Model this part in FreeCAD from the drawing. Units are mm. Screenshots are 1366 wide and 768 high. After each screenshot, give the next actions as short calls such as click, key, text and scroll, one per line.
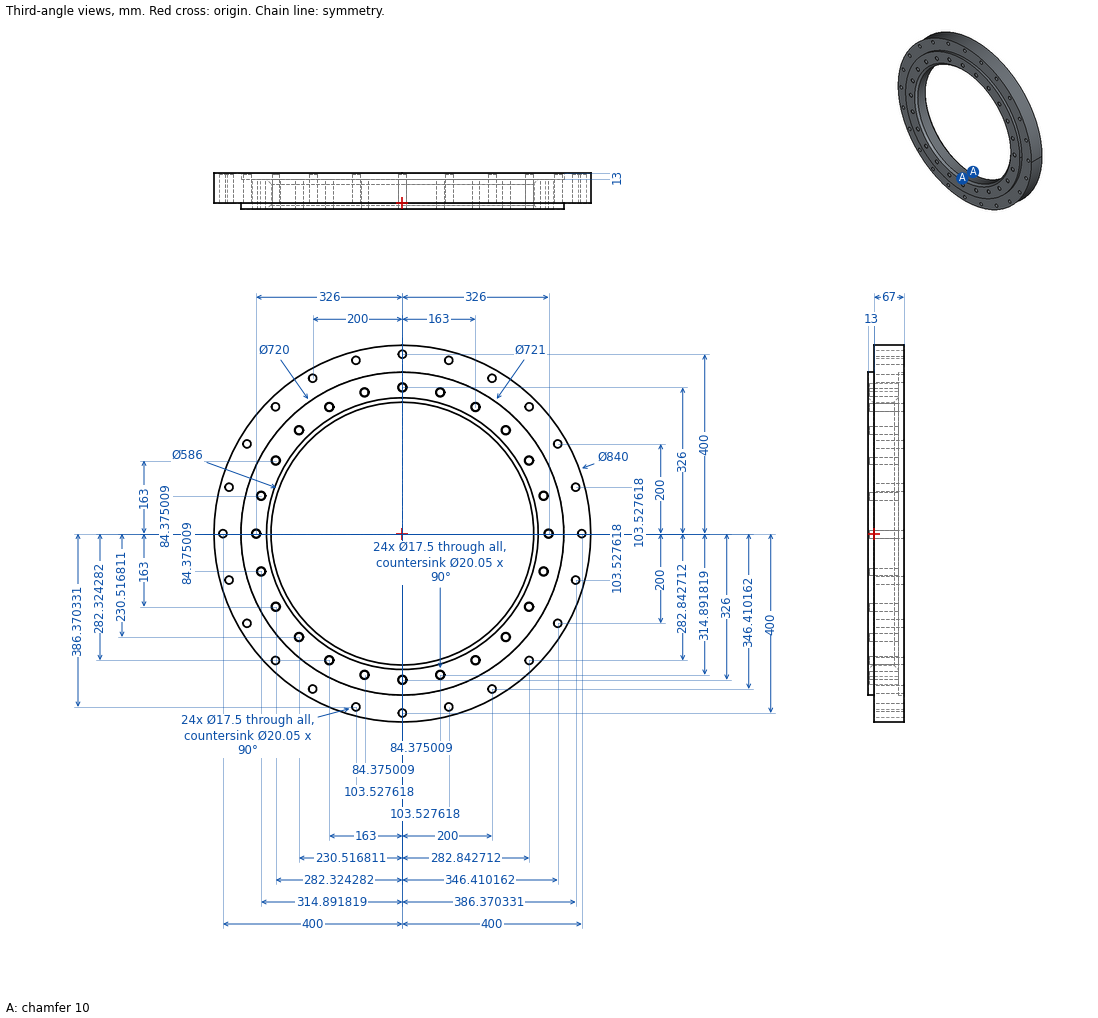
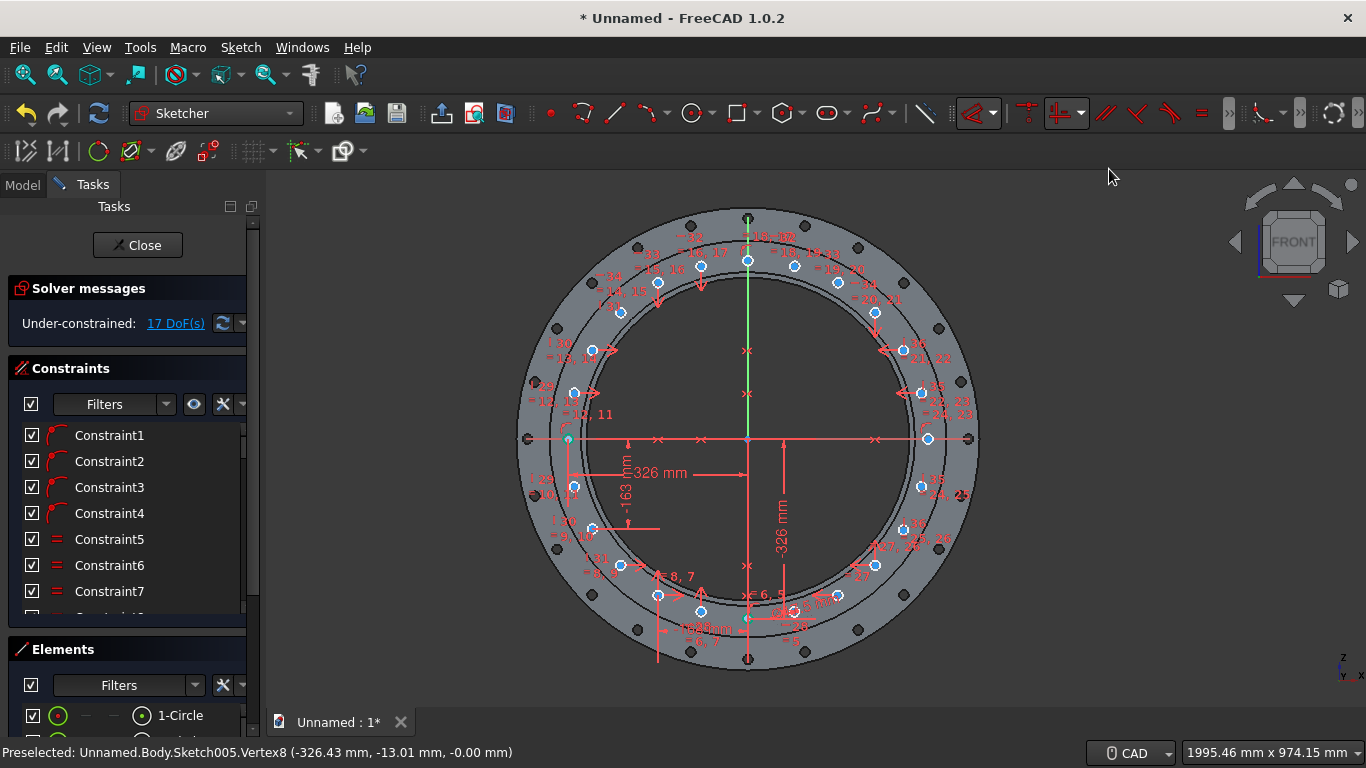
scroll(592, 350, up, 4)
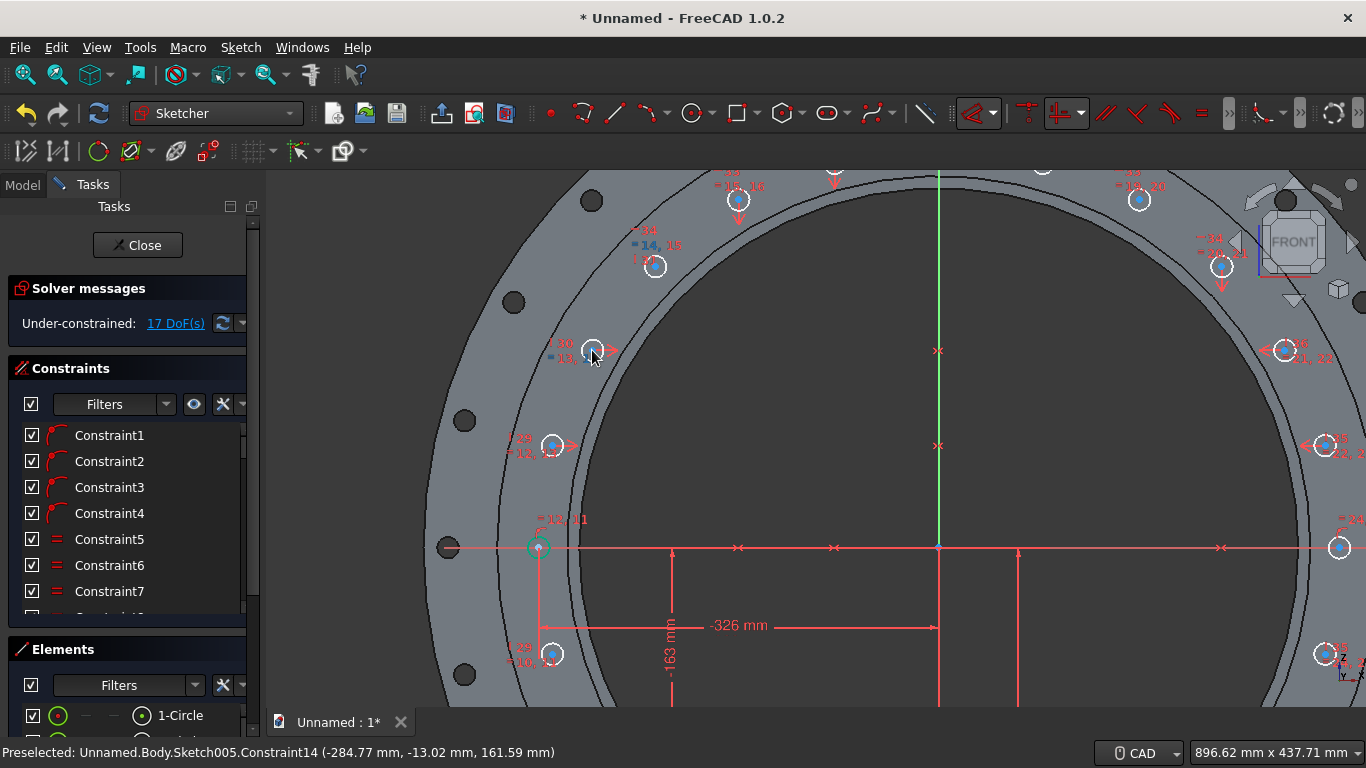
scroll(593, 350, up, 4)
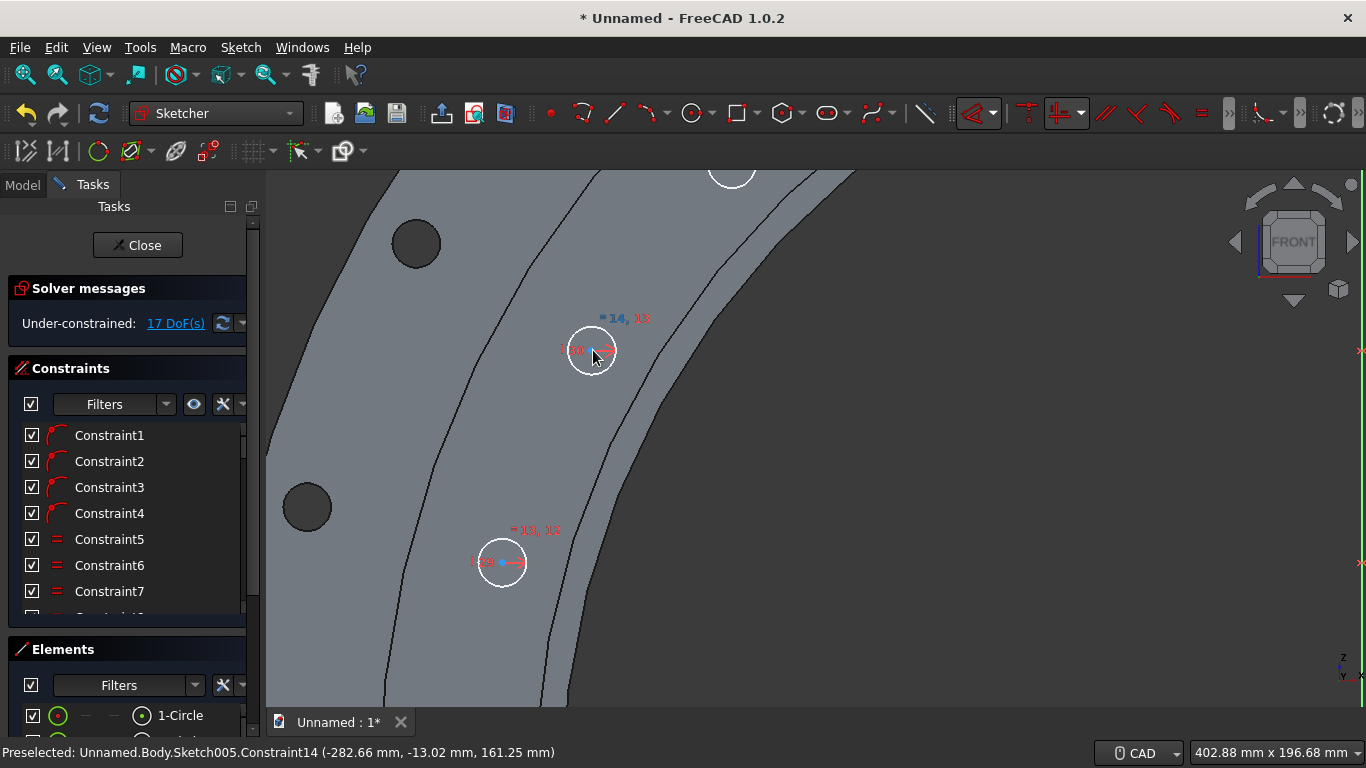
click(592, 351)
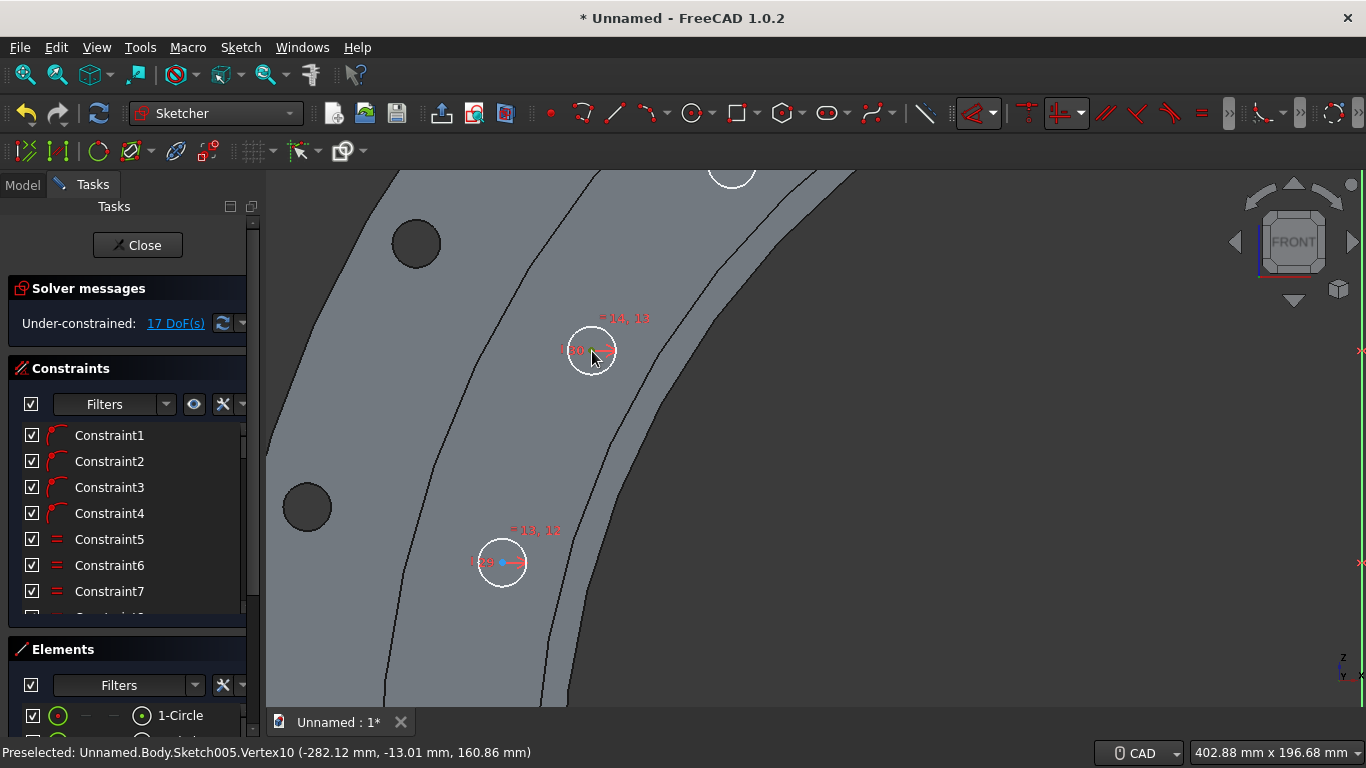
key(i)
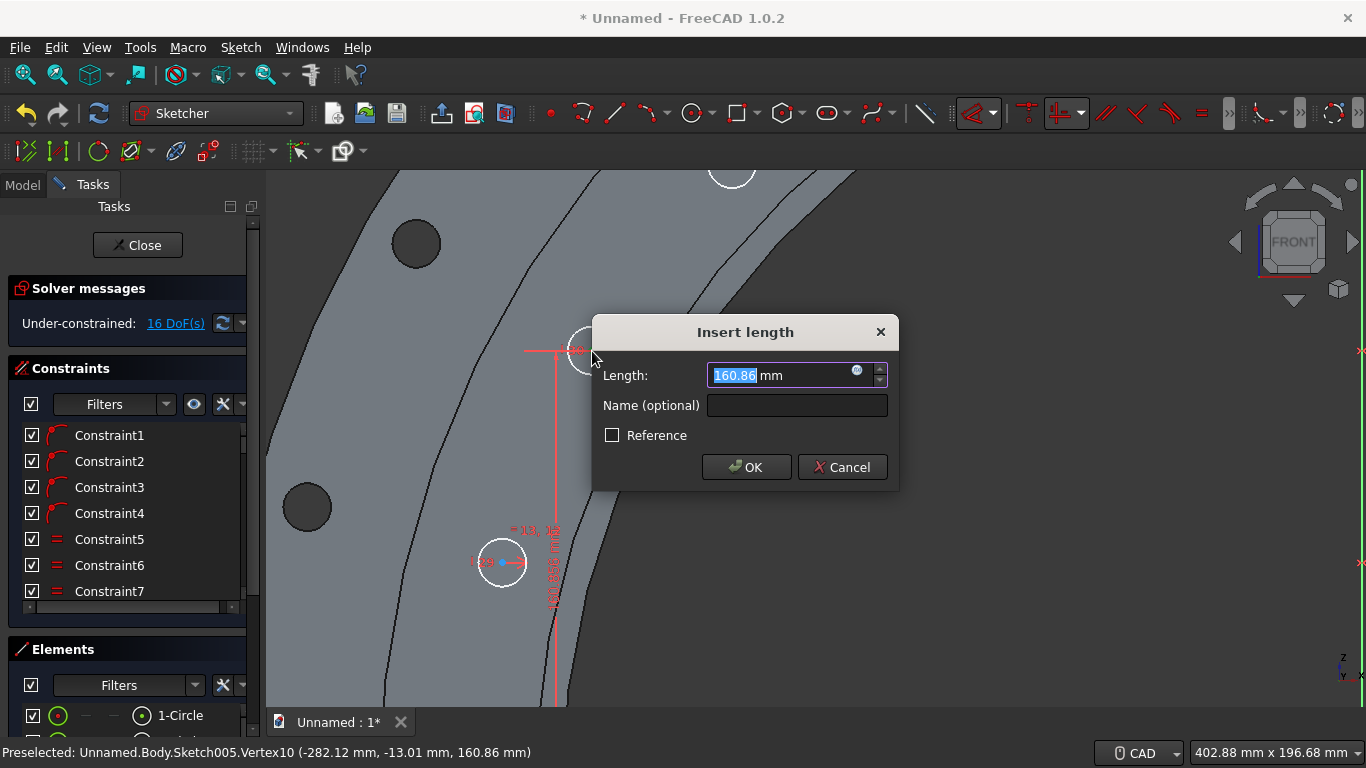
text(163)
key(Return)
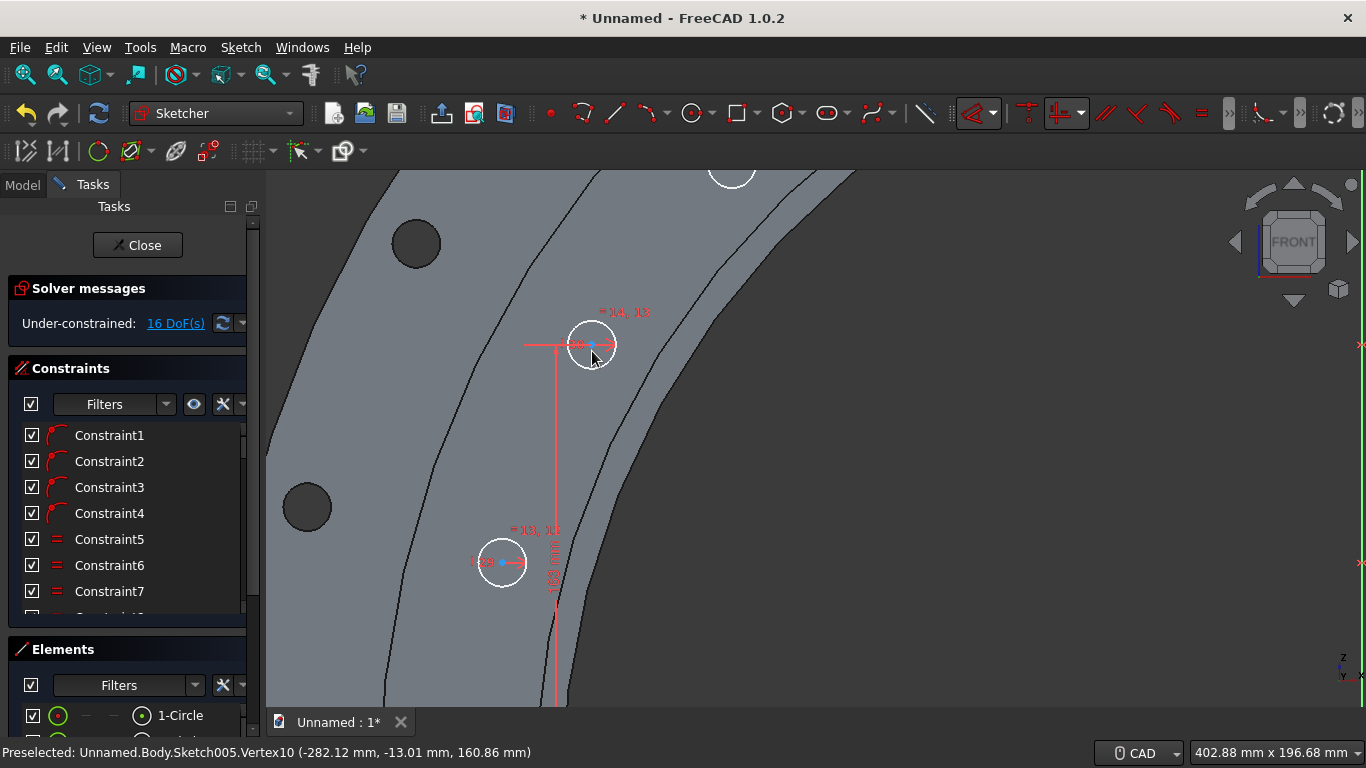
scroll(592, 350, down, 8)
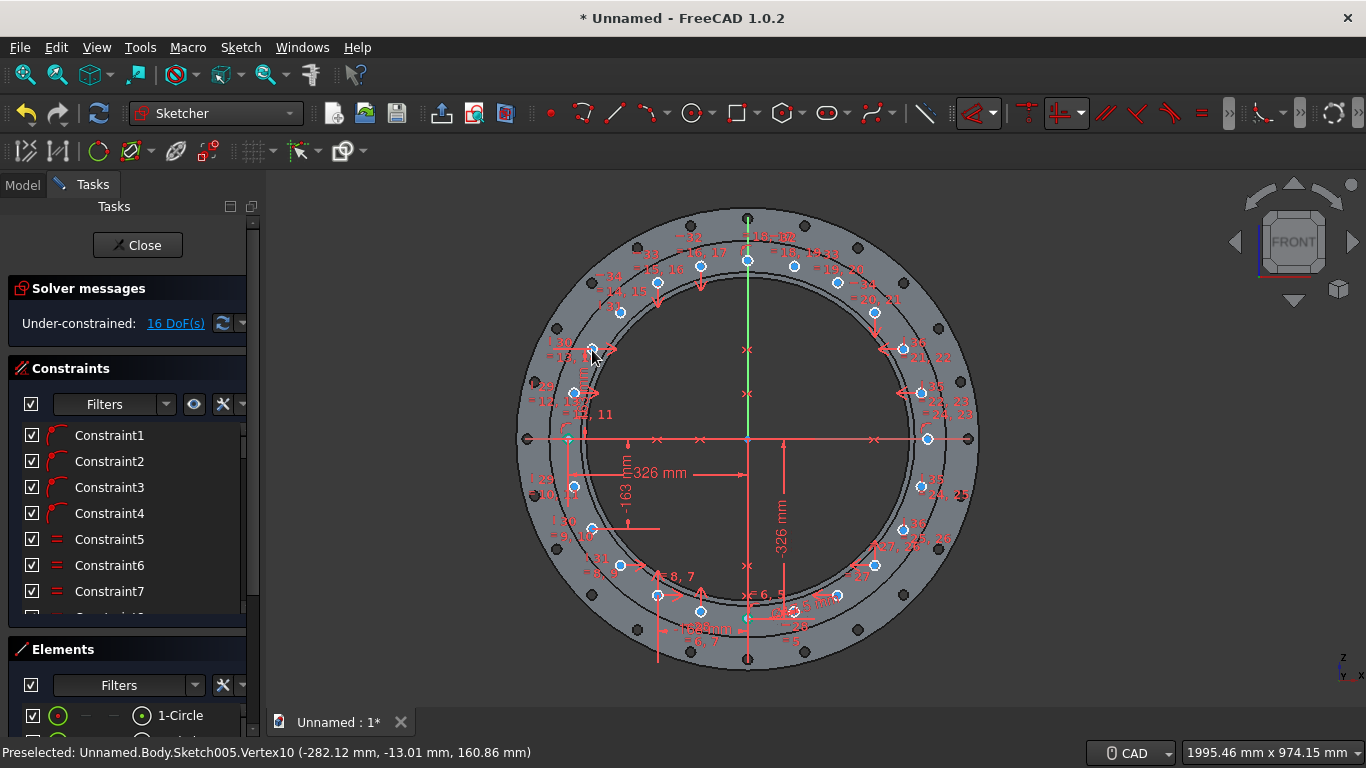
click(748, 261)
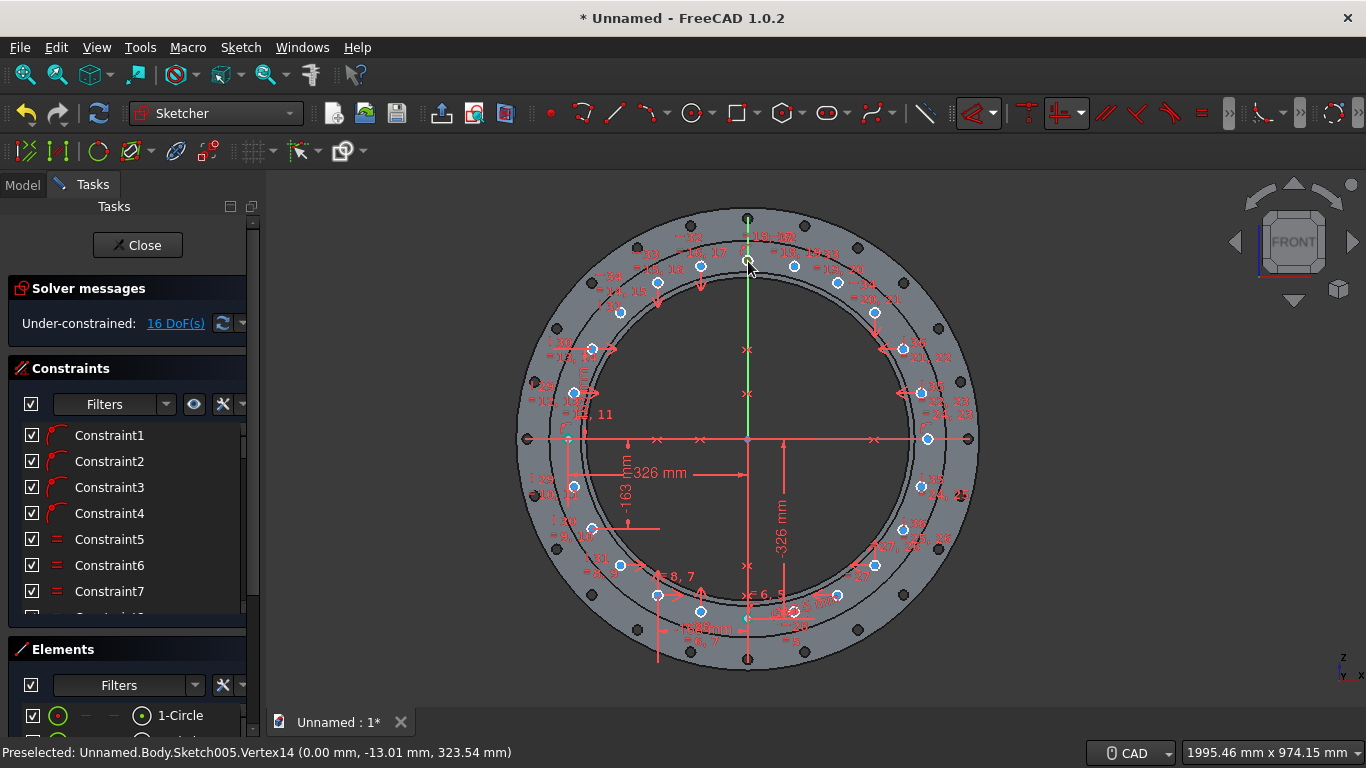
key(i)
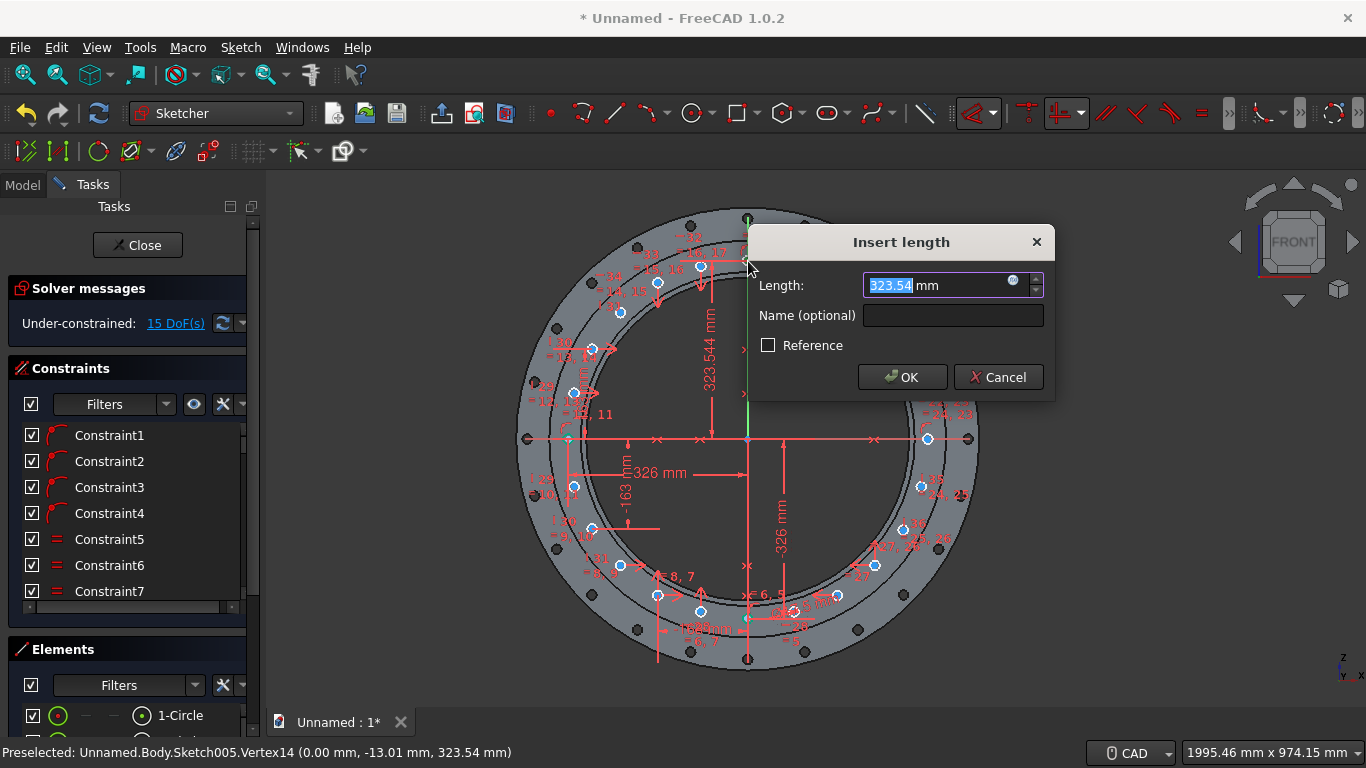
text(326)
key(Return)